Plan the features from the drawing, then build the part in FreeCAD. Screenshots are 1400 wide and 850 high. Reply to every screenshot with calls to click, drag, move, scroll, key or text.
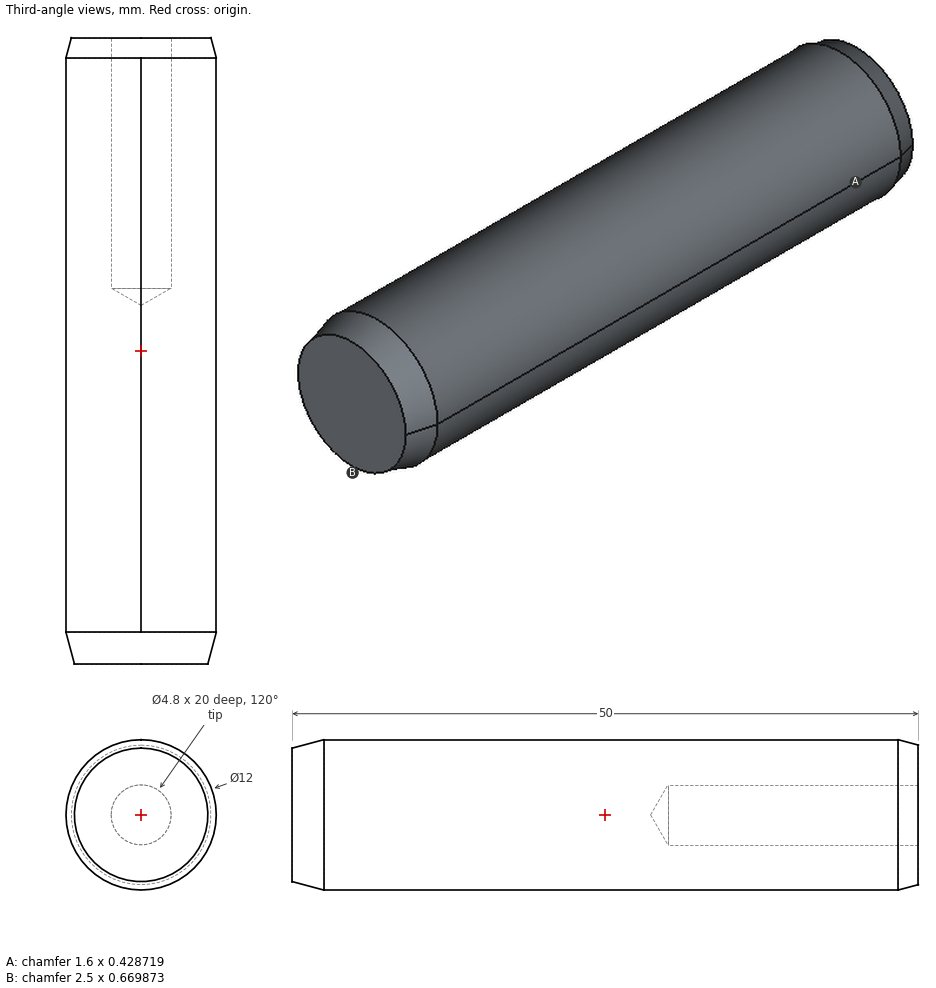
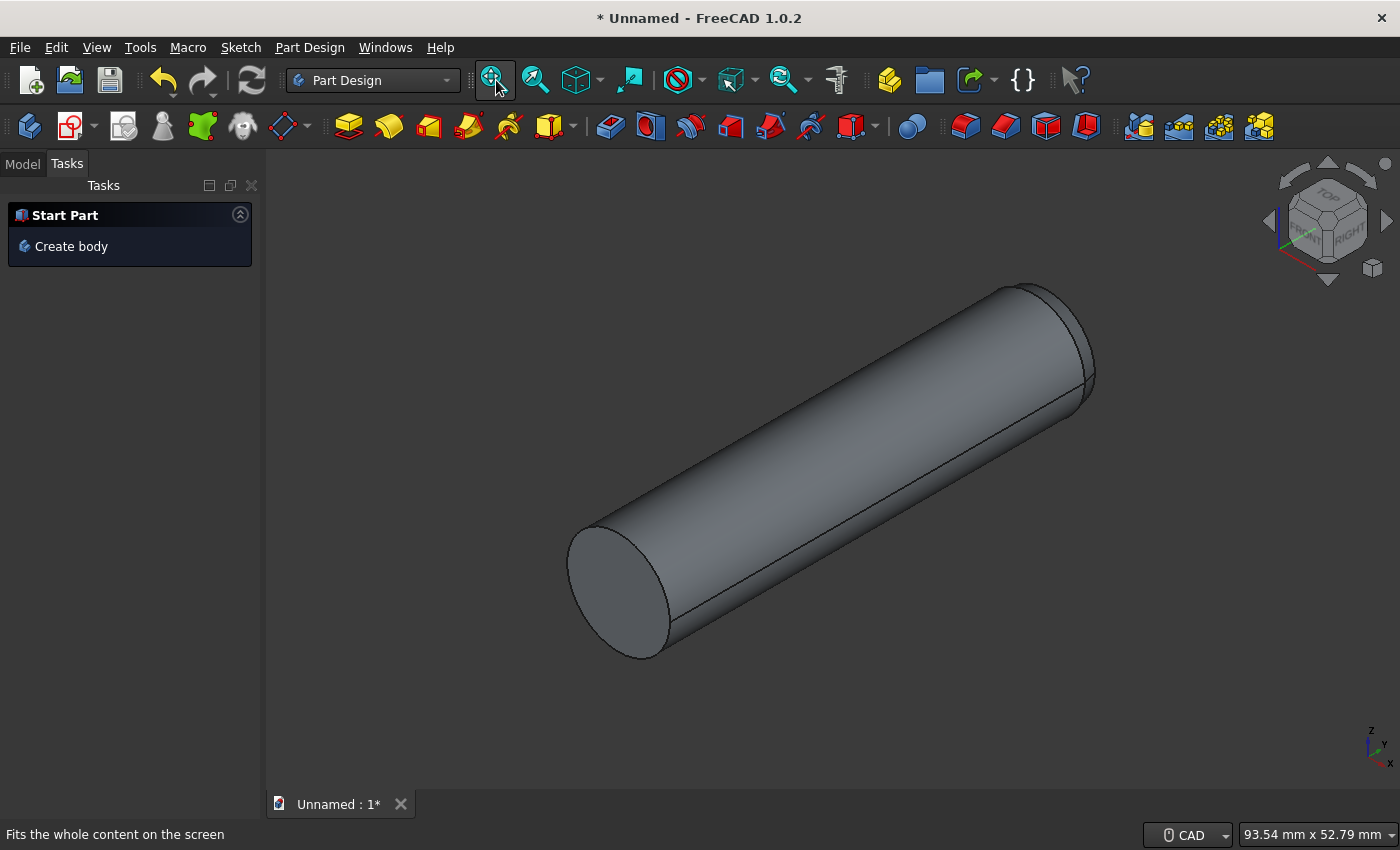
click(603, 526)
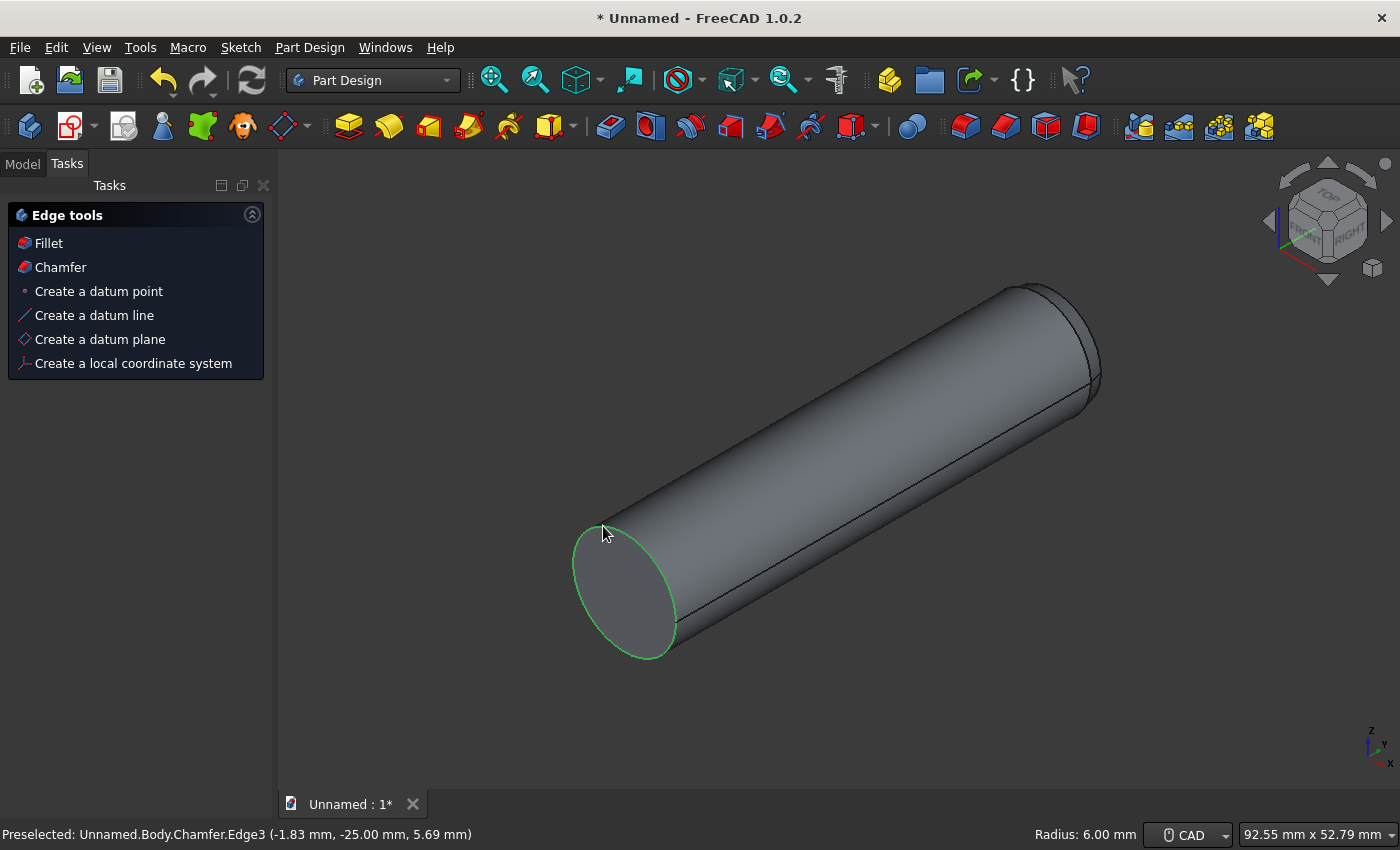
click(1006, 126)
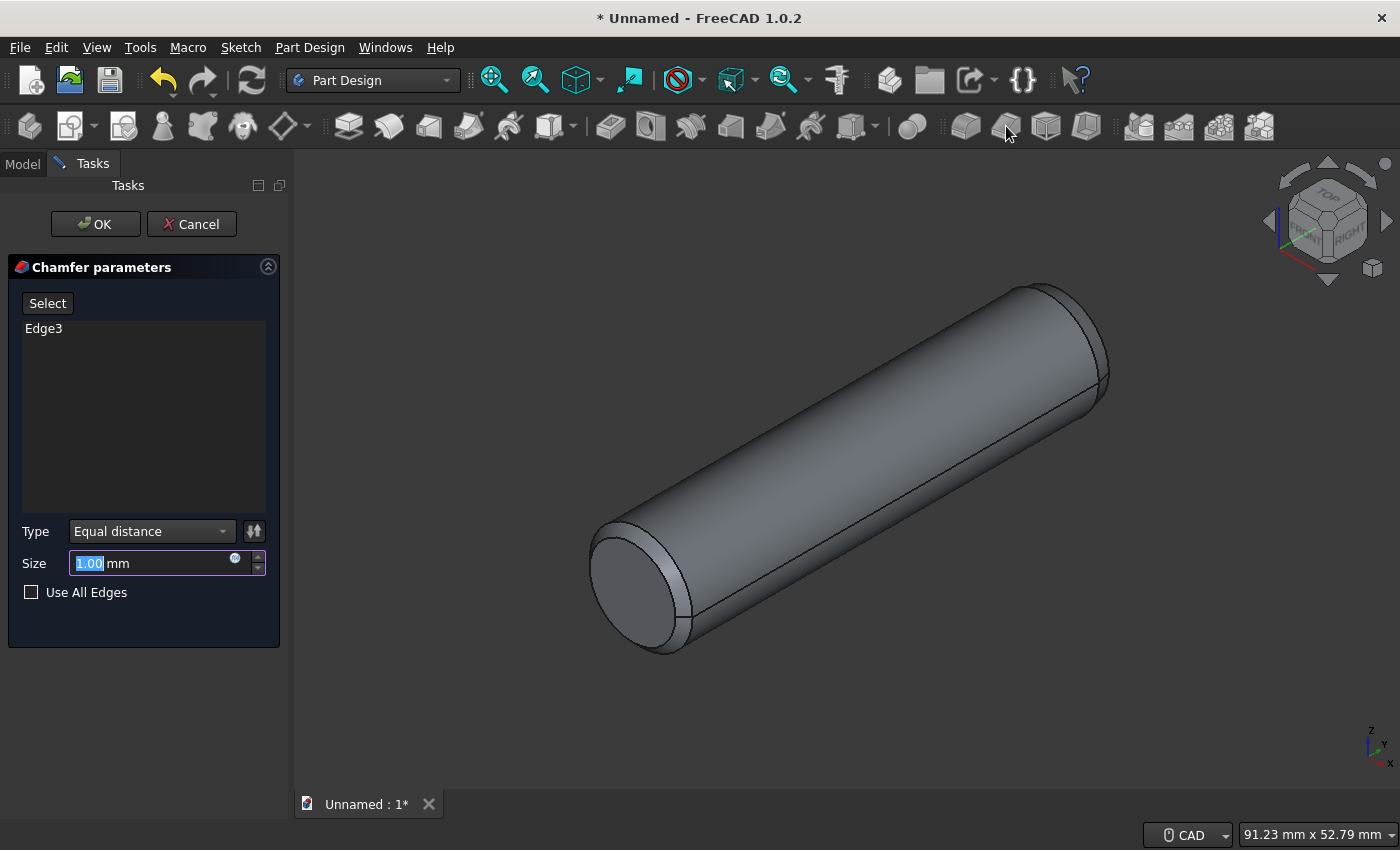
text(2.5)
key(Tab)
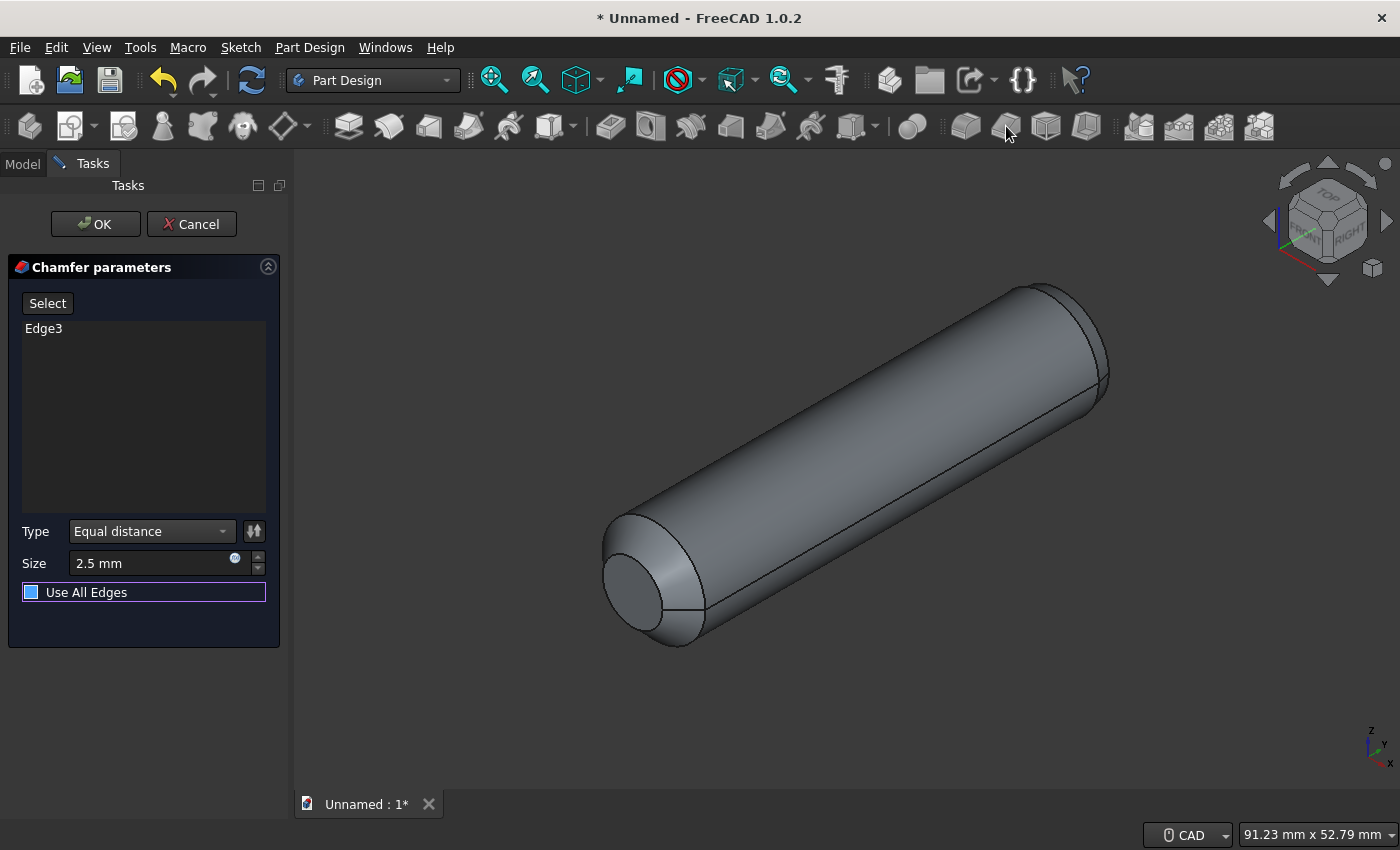
click(153, 532)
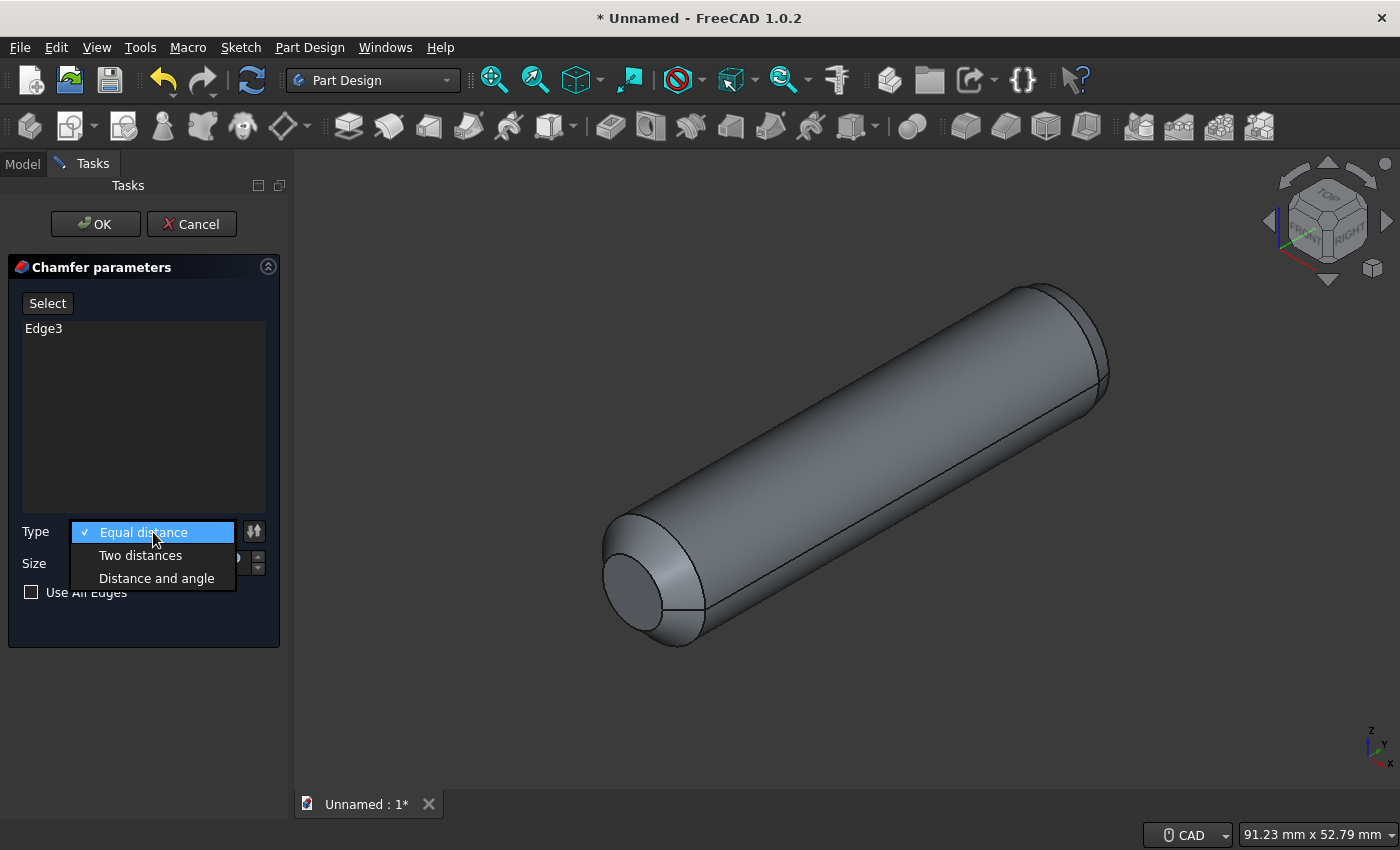
click(152, 556)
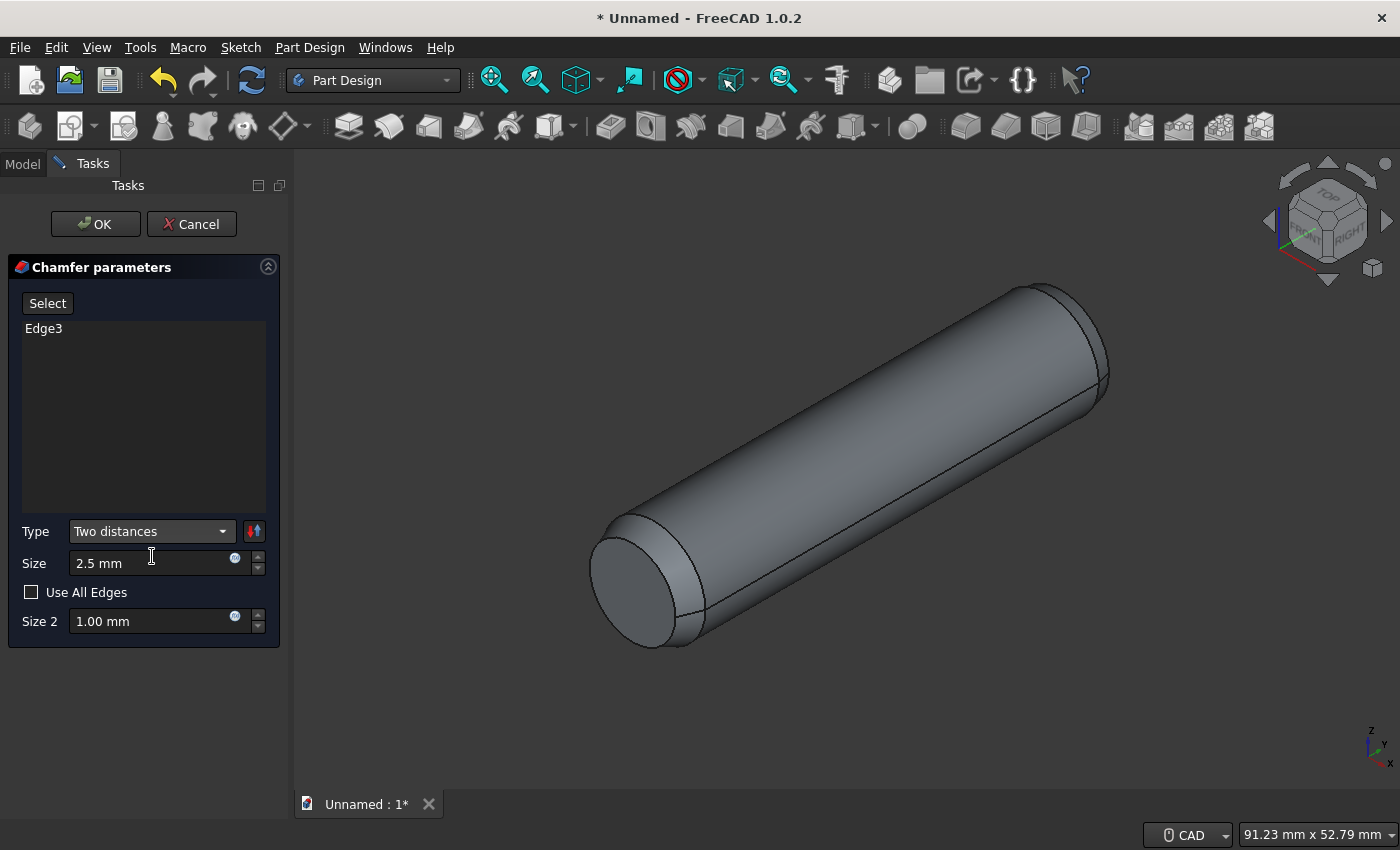
triple_click(160, 621)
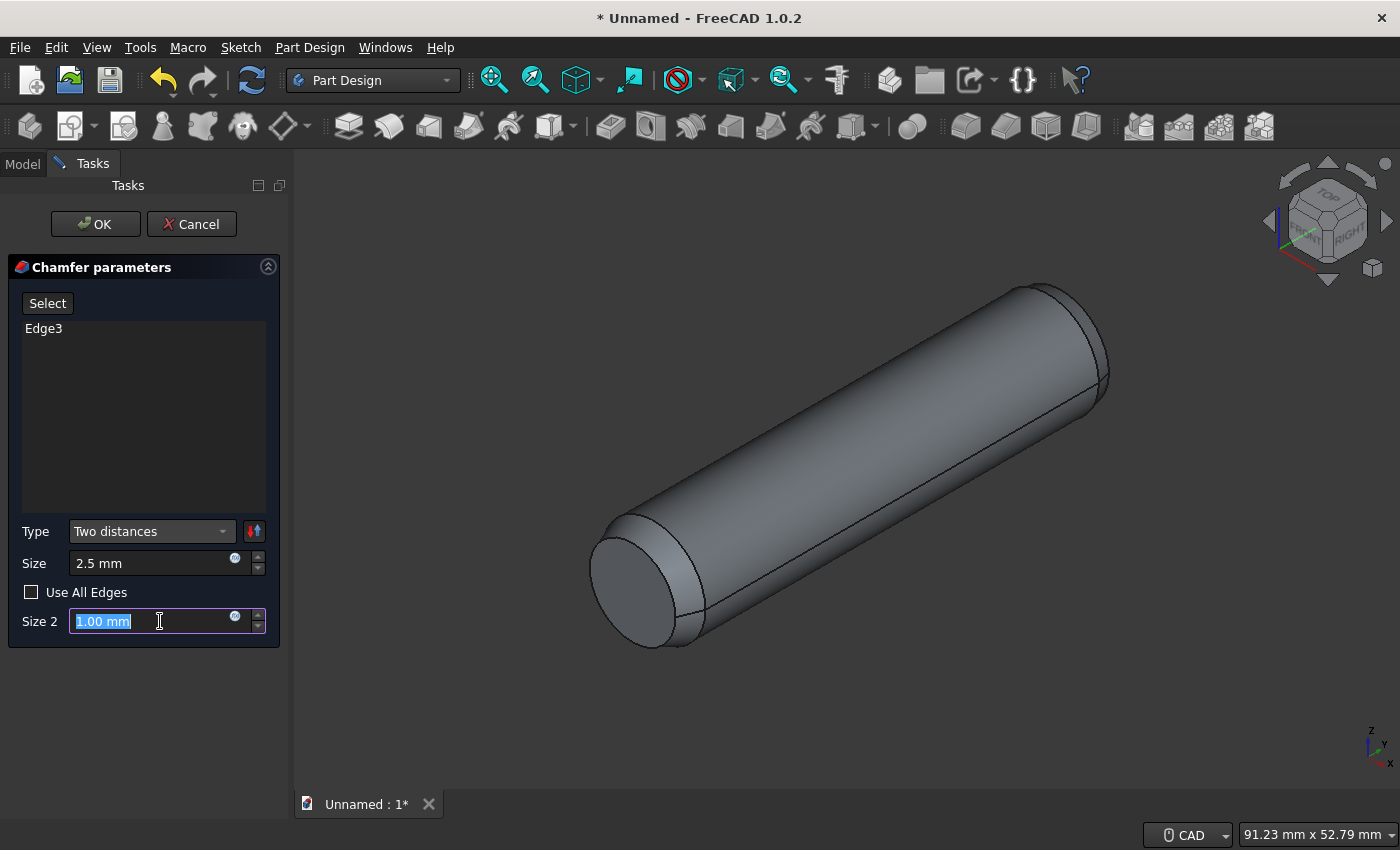
text(0.669873)
key(Tab)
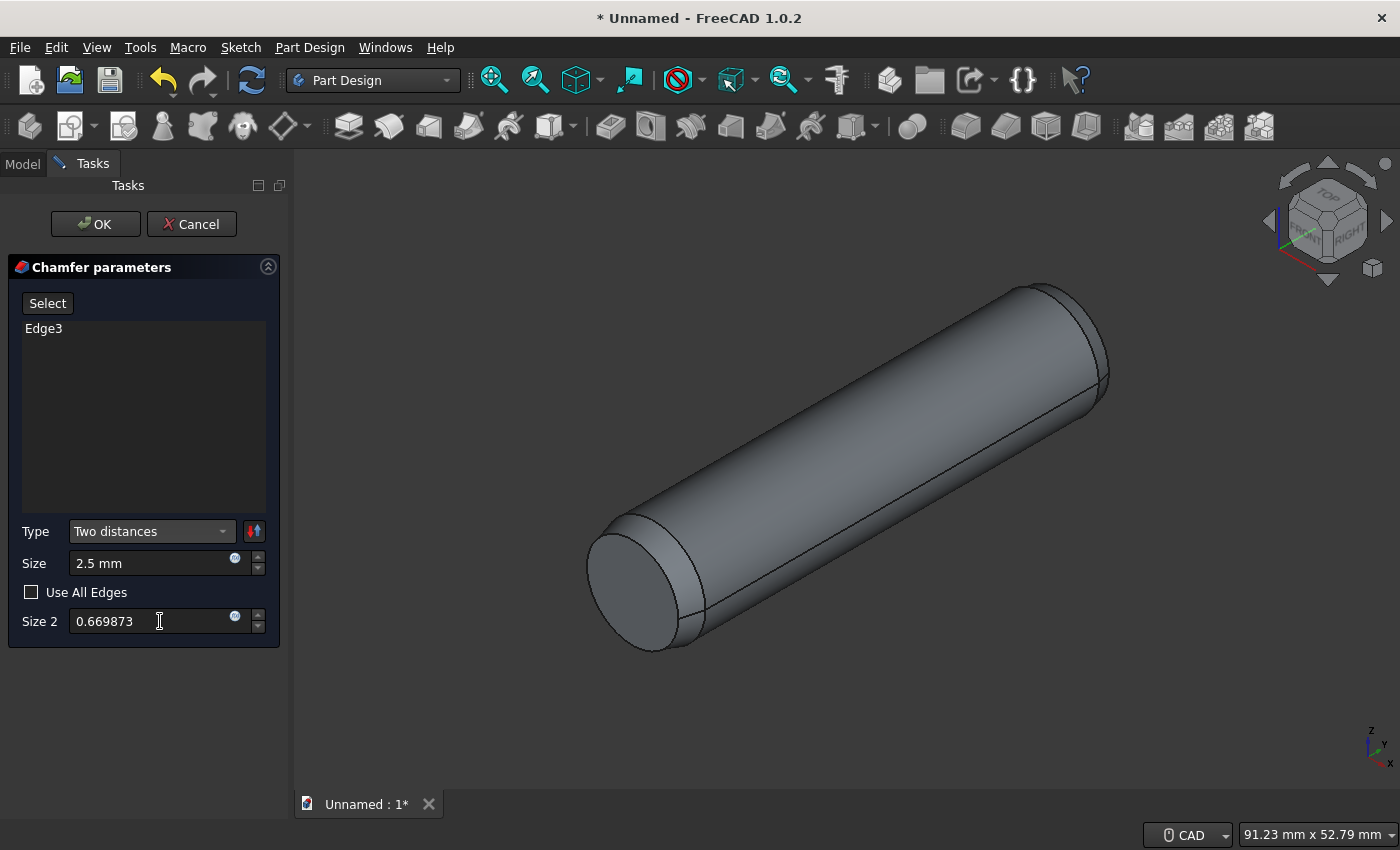
click(96, 224)